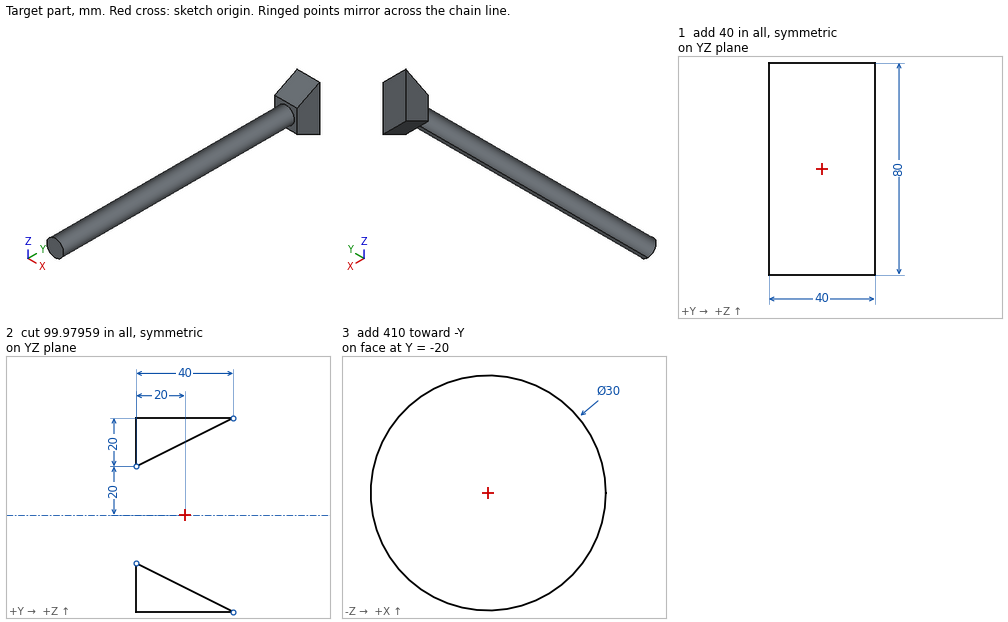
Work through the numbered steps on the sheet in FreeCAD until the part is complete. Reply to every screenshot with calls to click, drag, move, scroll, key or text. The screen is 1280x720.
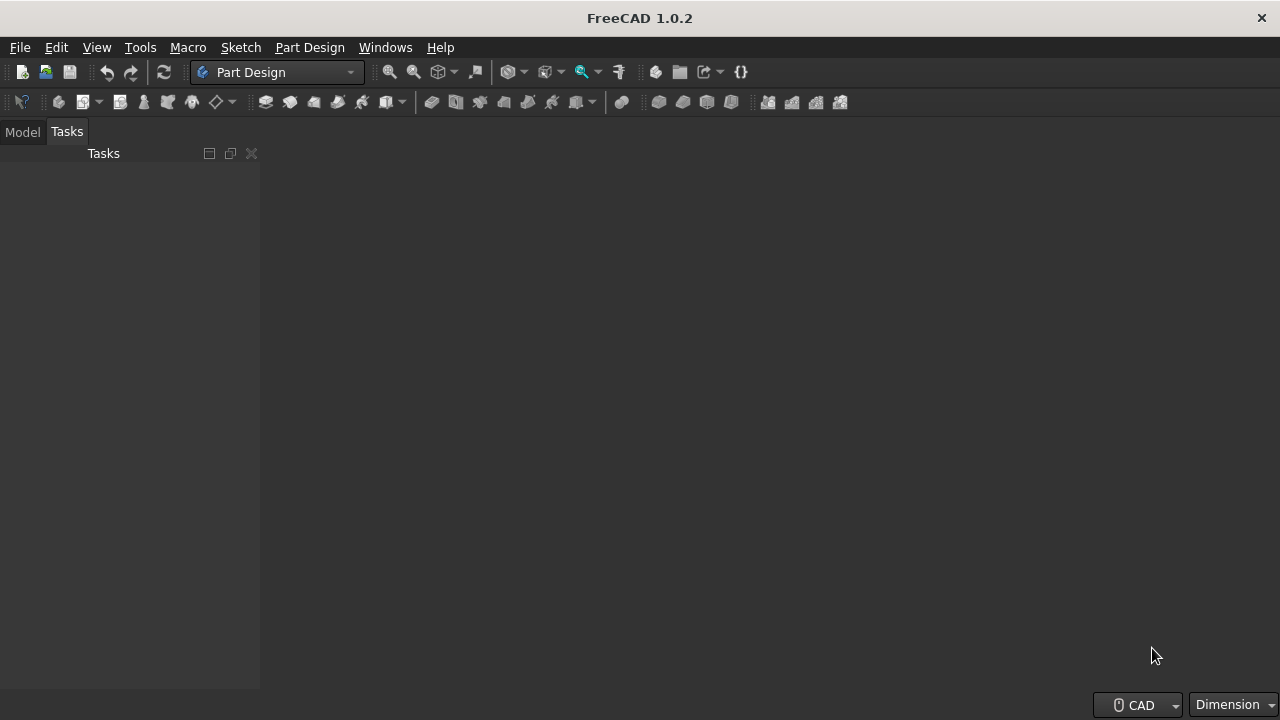
key(ctrl+n)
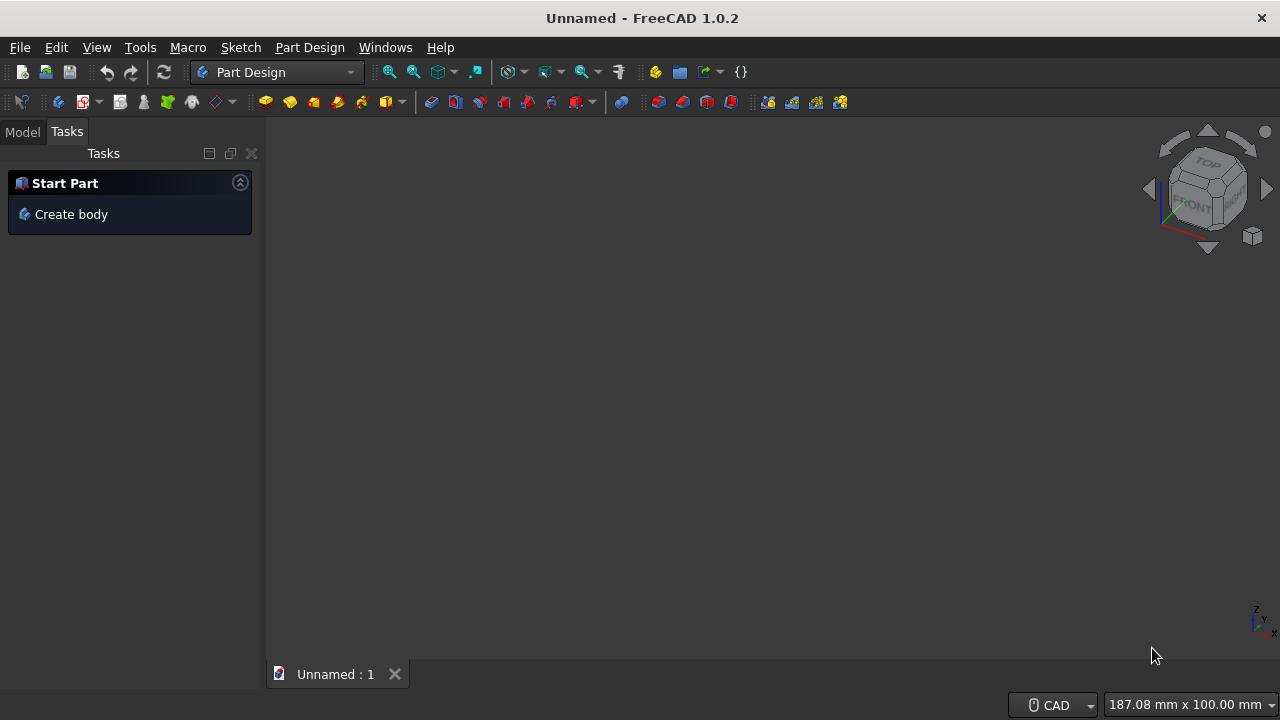
click(84, 102)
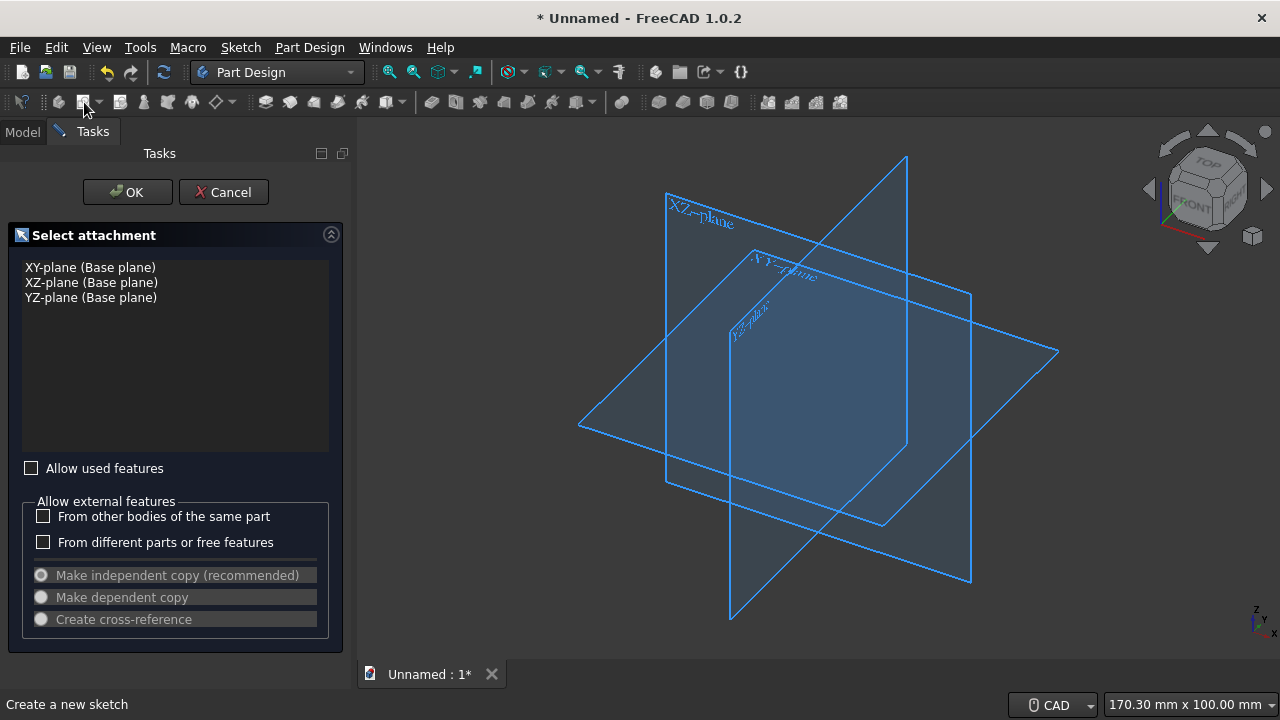
click(82, 298)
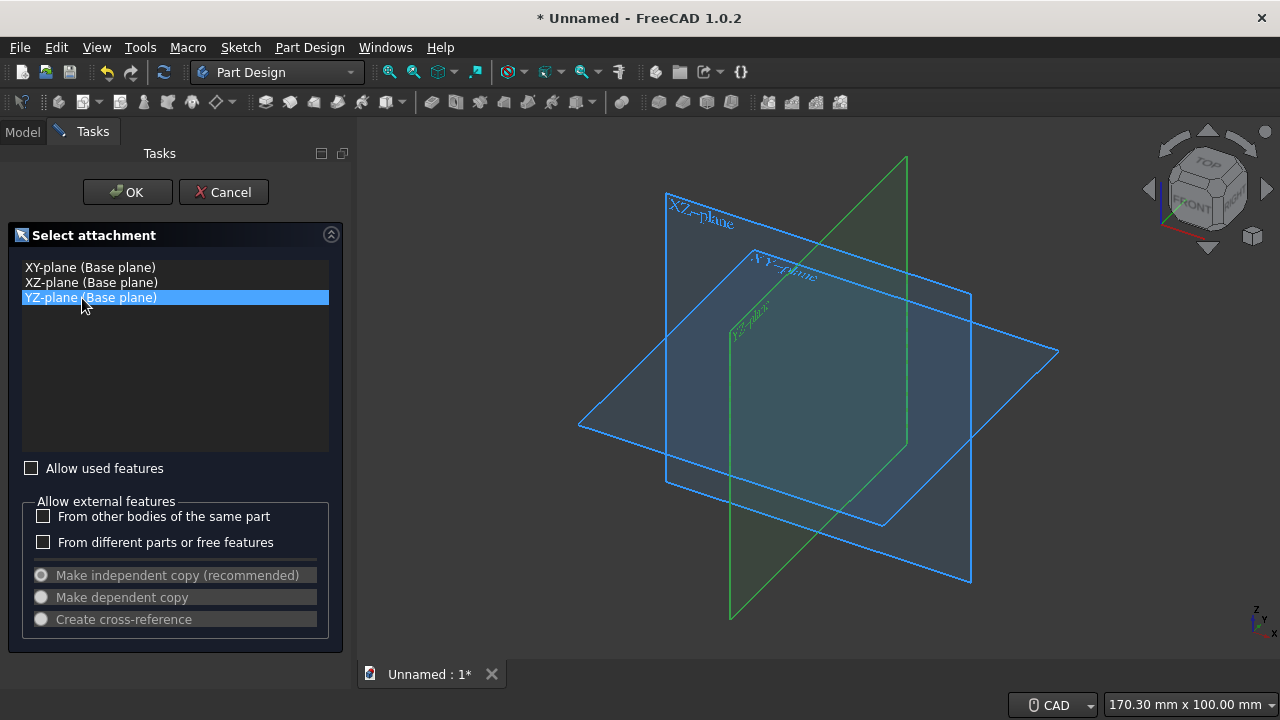
click(128, 192)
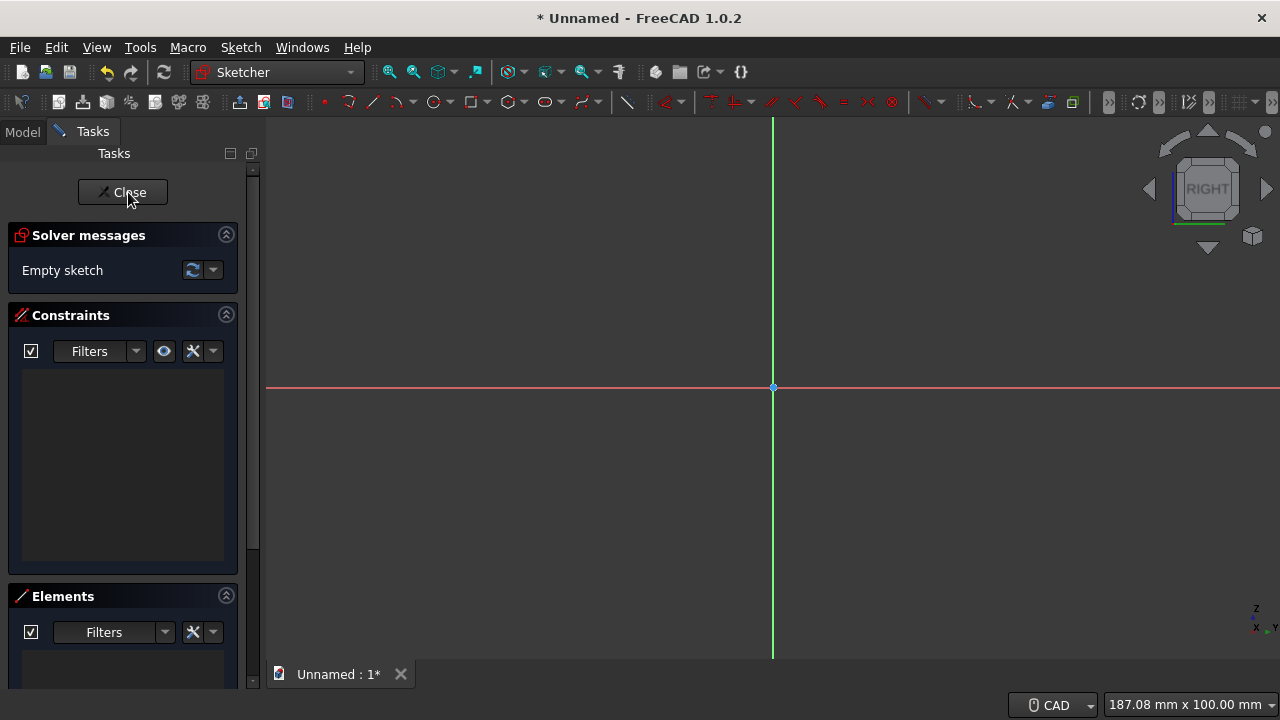
key(g)
key(v)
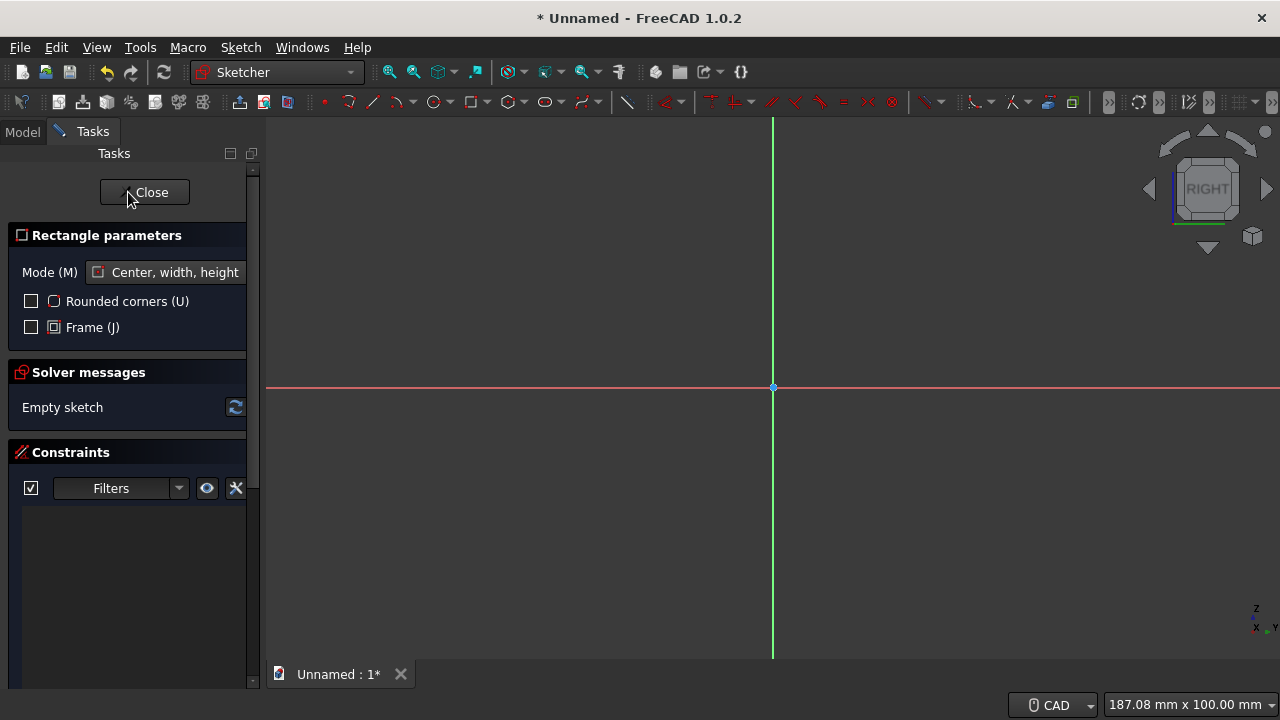
click(773, 388)
click(881, 171)
key(Escape)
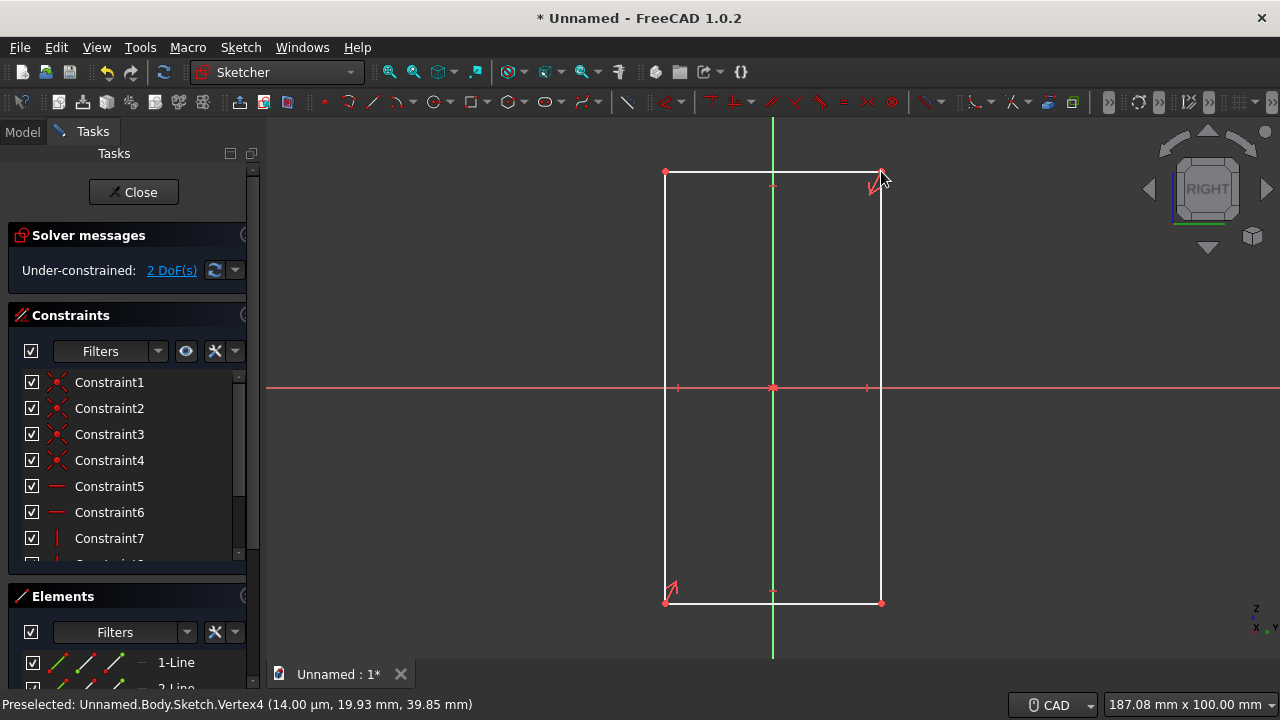
click(730, 604)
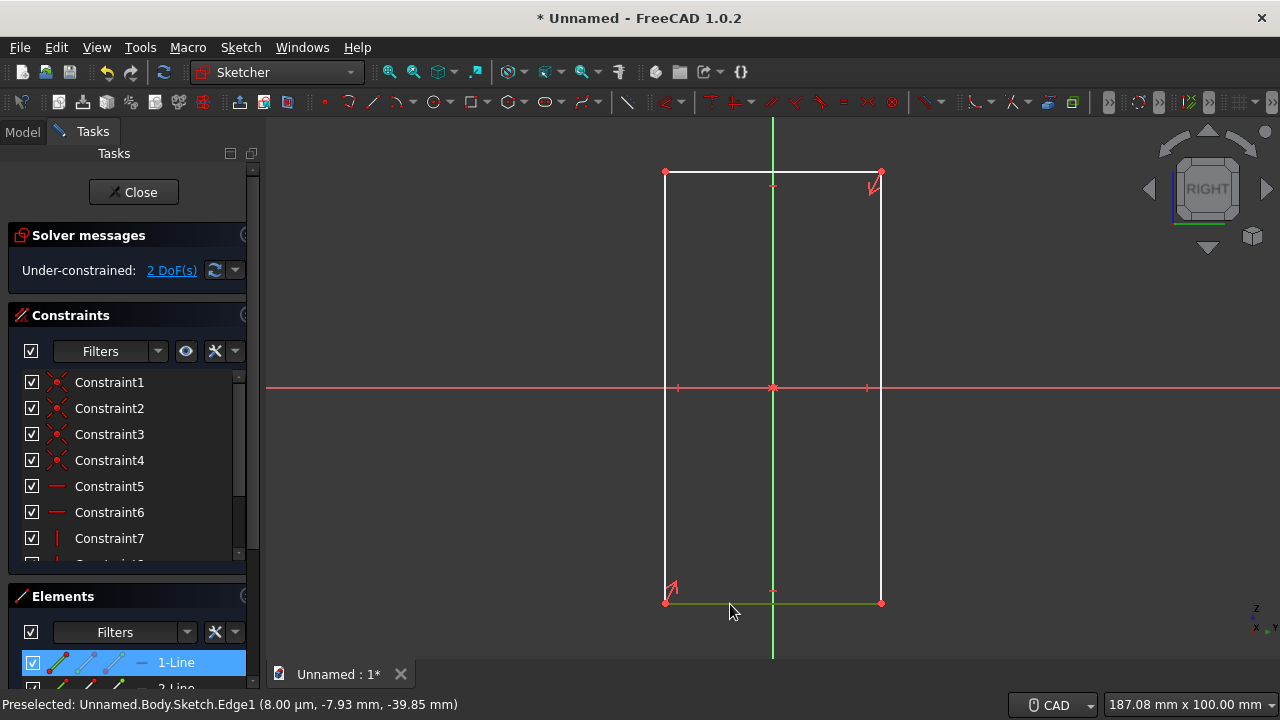
key(l)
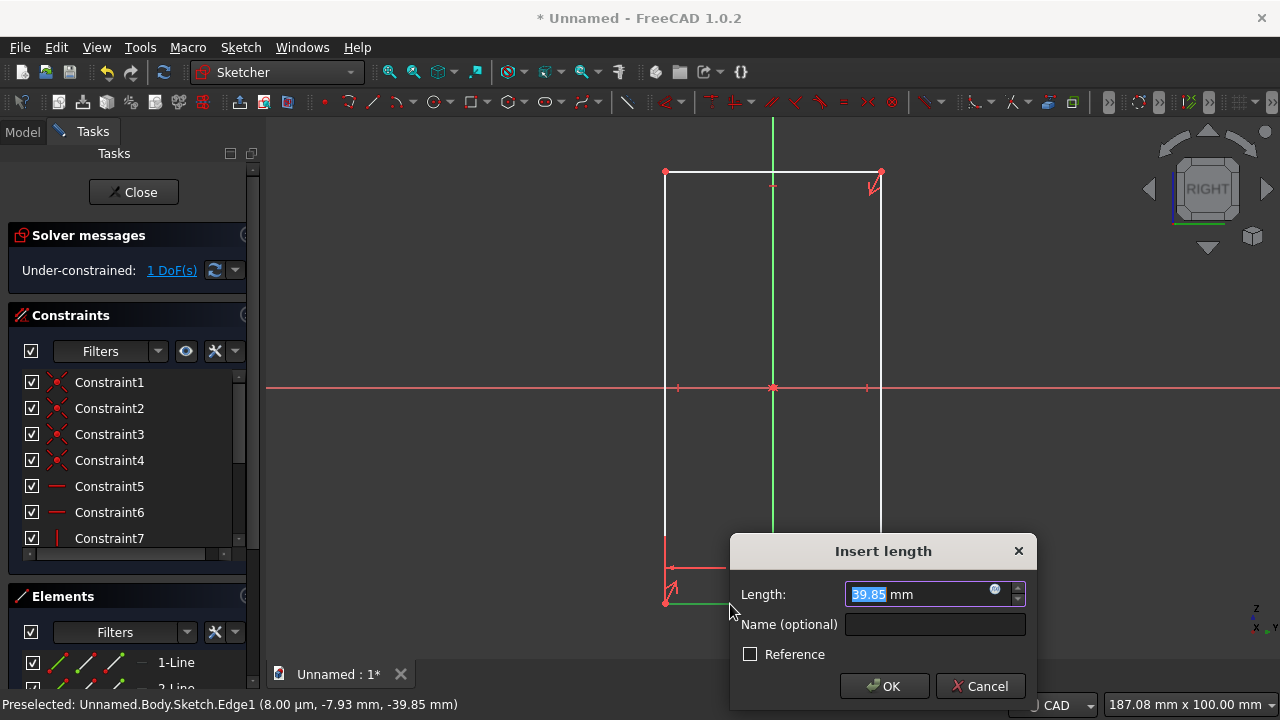
text(40)
key(Return)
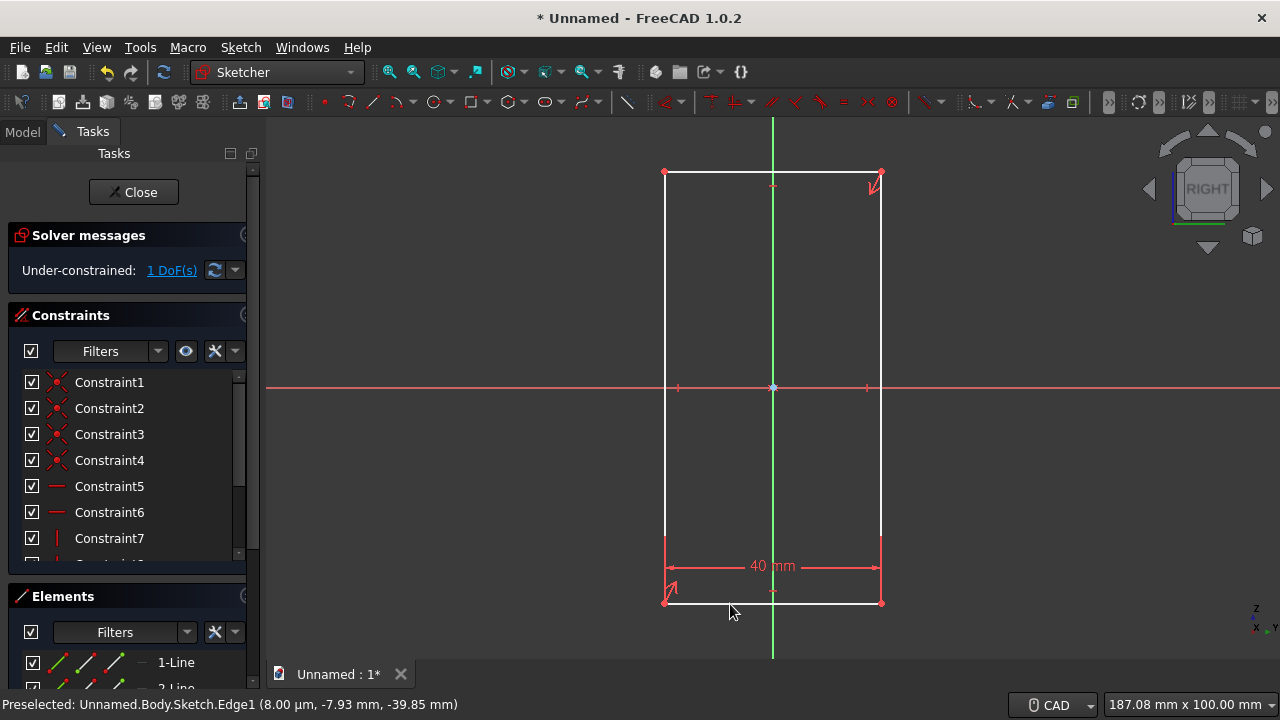
click(881, 474)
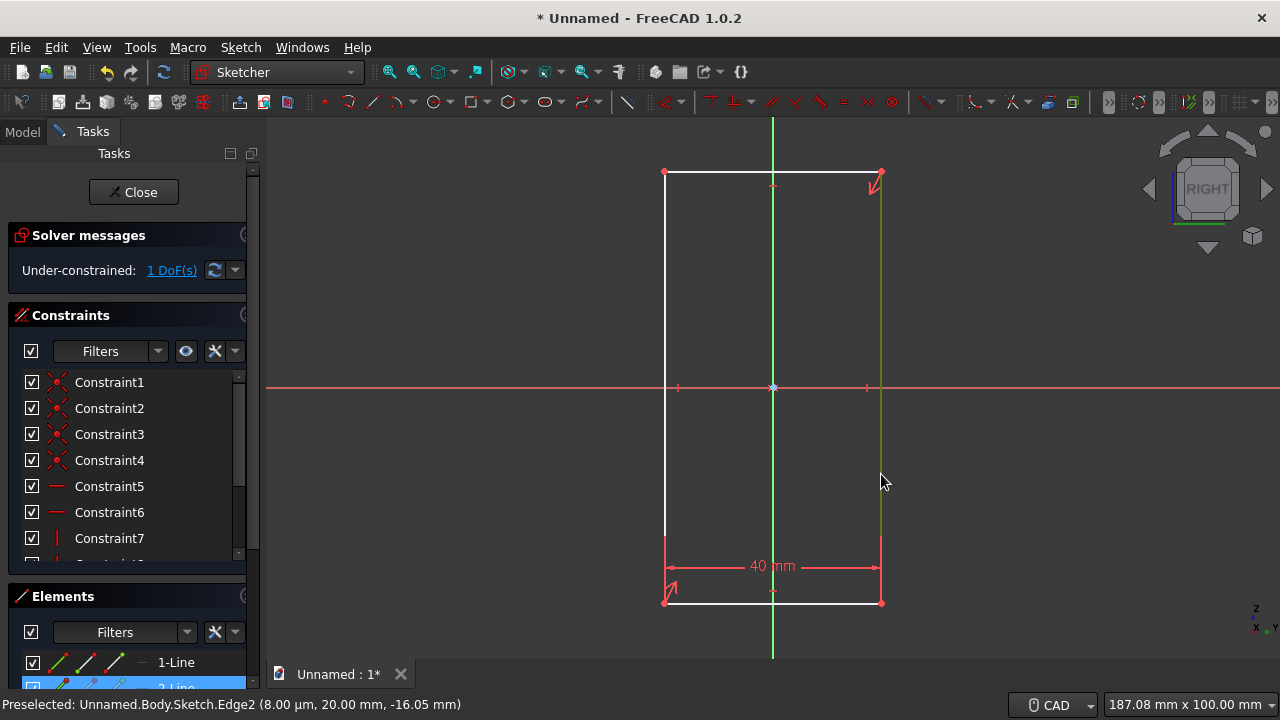
key(i)